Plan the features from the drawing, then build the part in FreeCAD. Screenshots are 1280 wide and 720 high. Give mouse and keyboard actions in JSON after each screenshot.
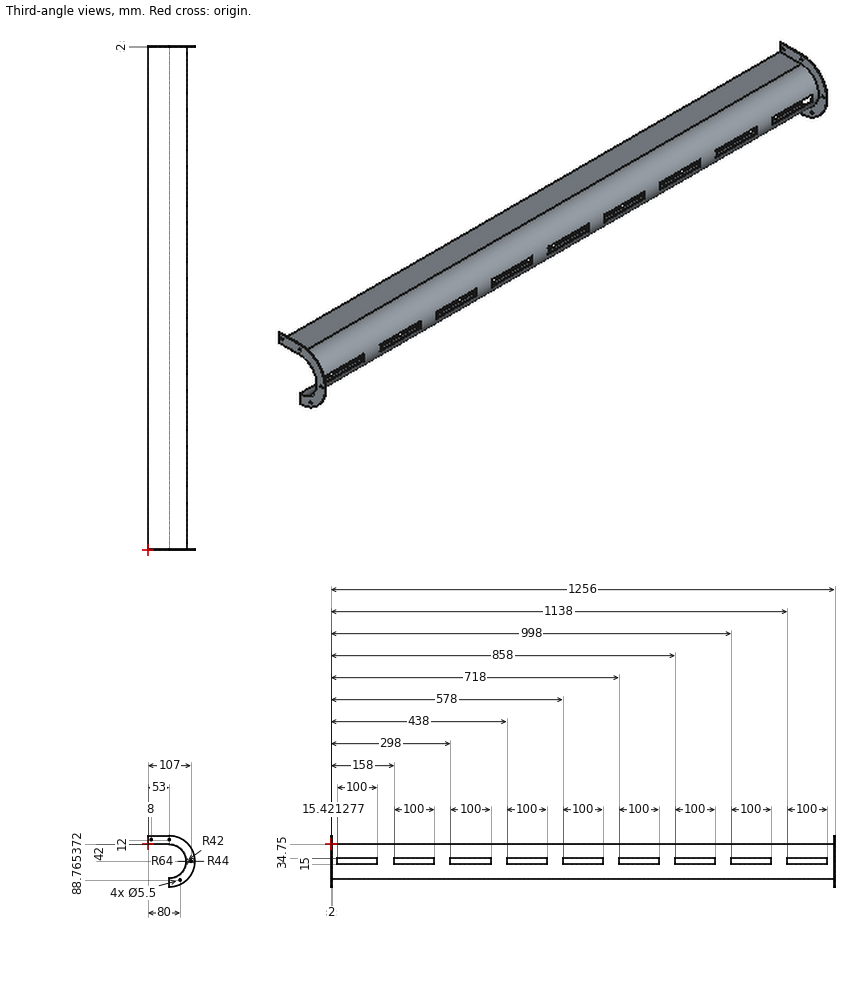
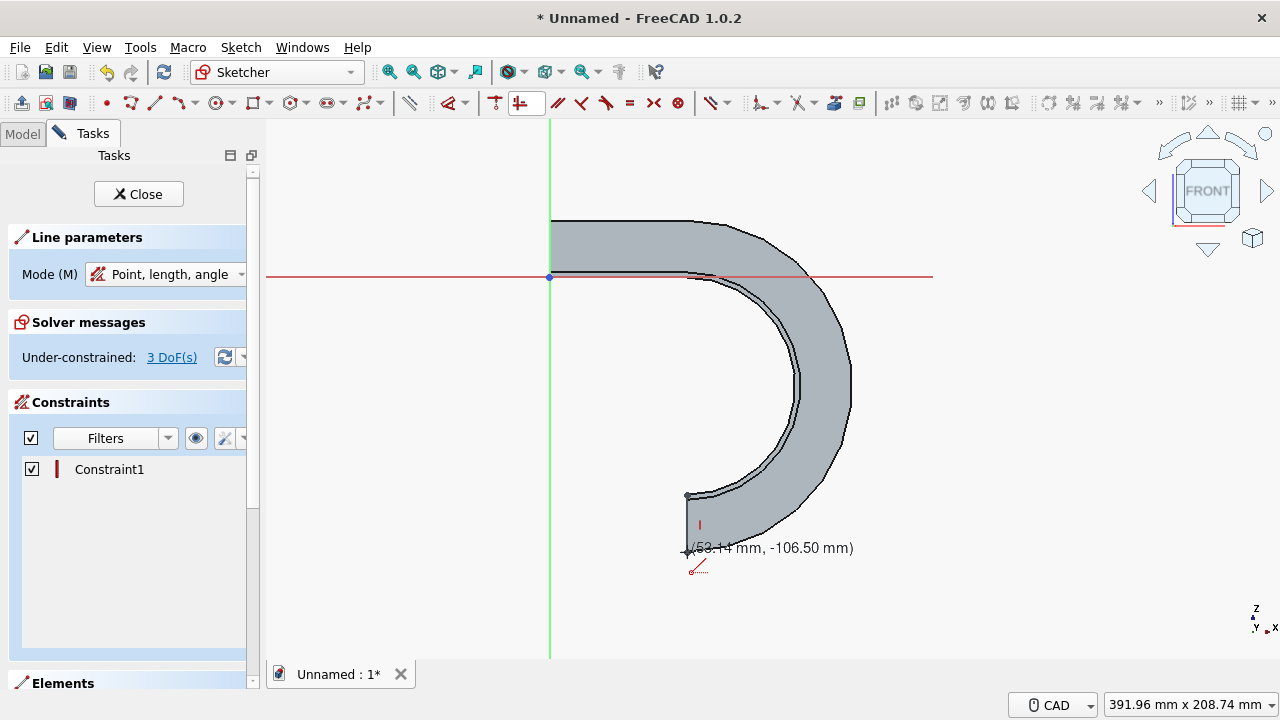
{"action": "left_click", "coordinate": [132, 104]}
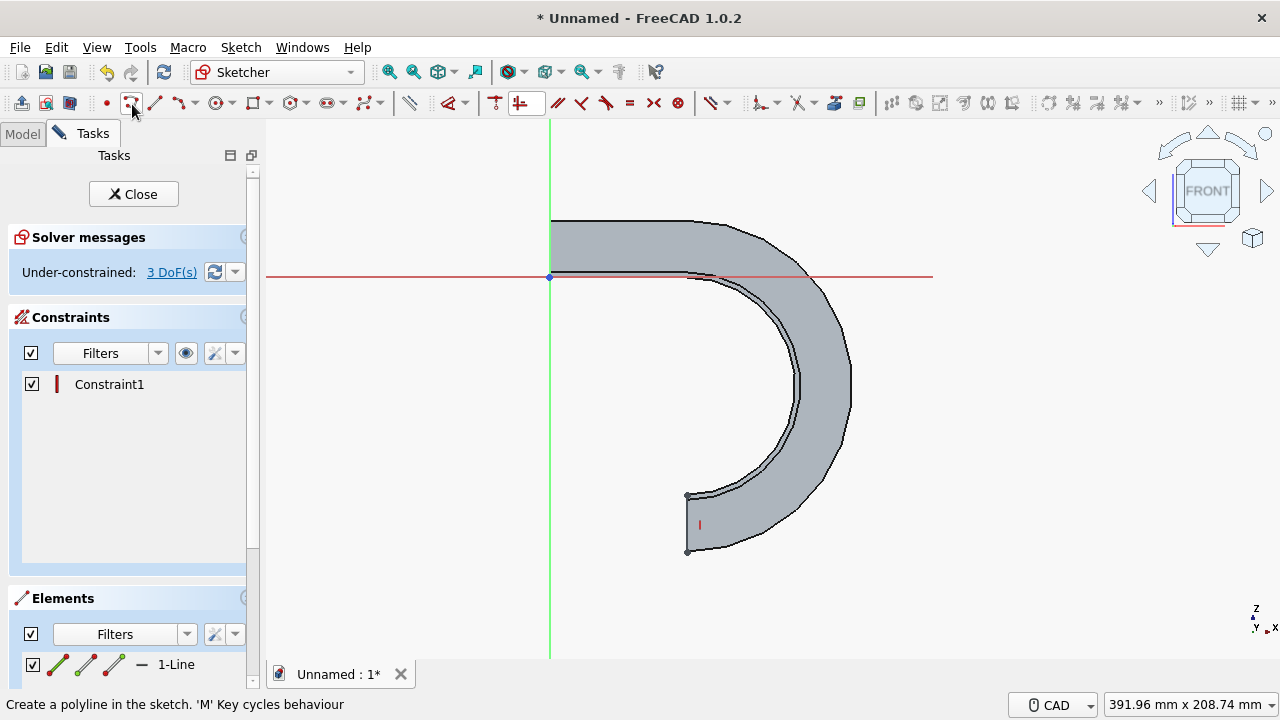
{"action": "left_click", "coordinate": [687, 221]}
{"action": "left_click", "coordinate": [550, 221]}
{"action": "left_click", "coordinate": [550, 277]}
{"action": "left_click", "coordinate": [687, 286]}
{"action": "right_click", "coordinate": [687, 286]}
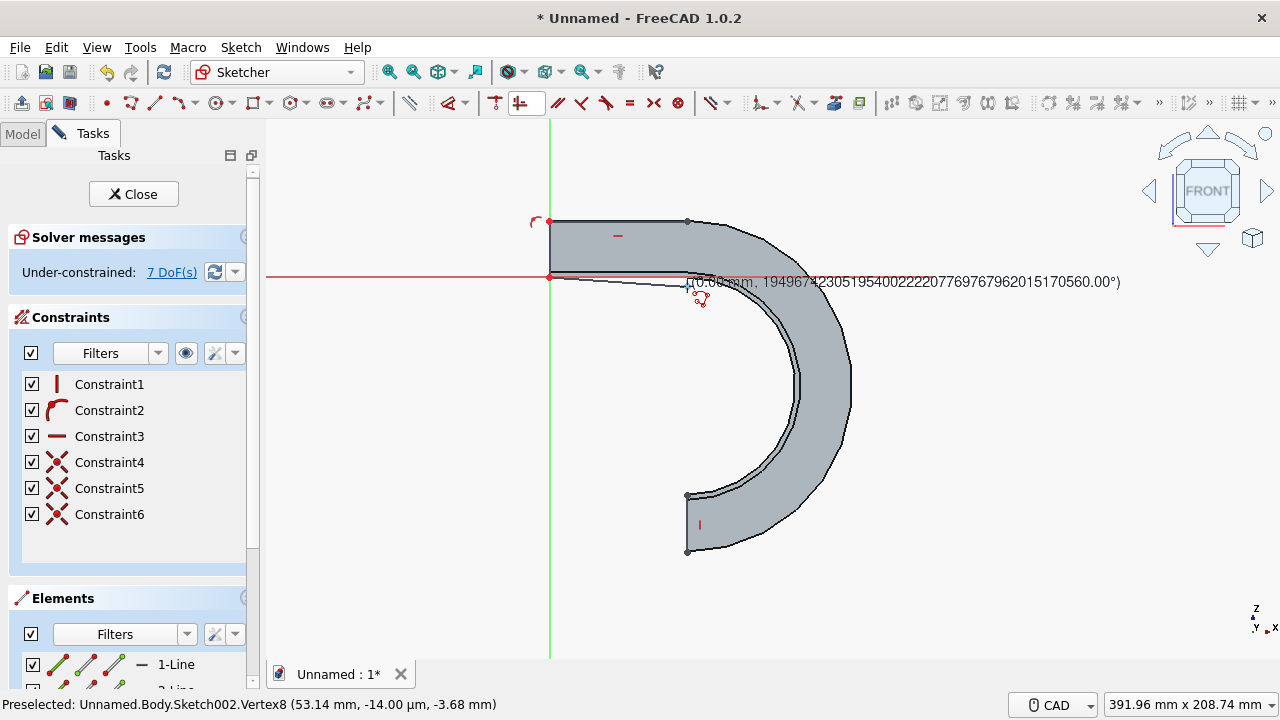
{"action": "left_click", "coordinate": [180, 104]}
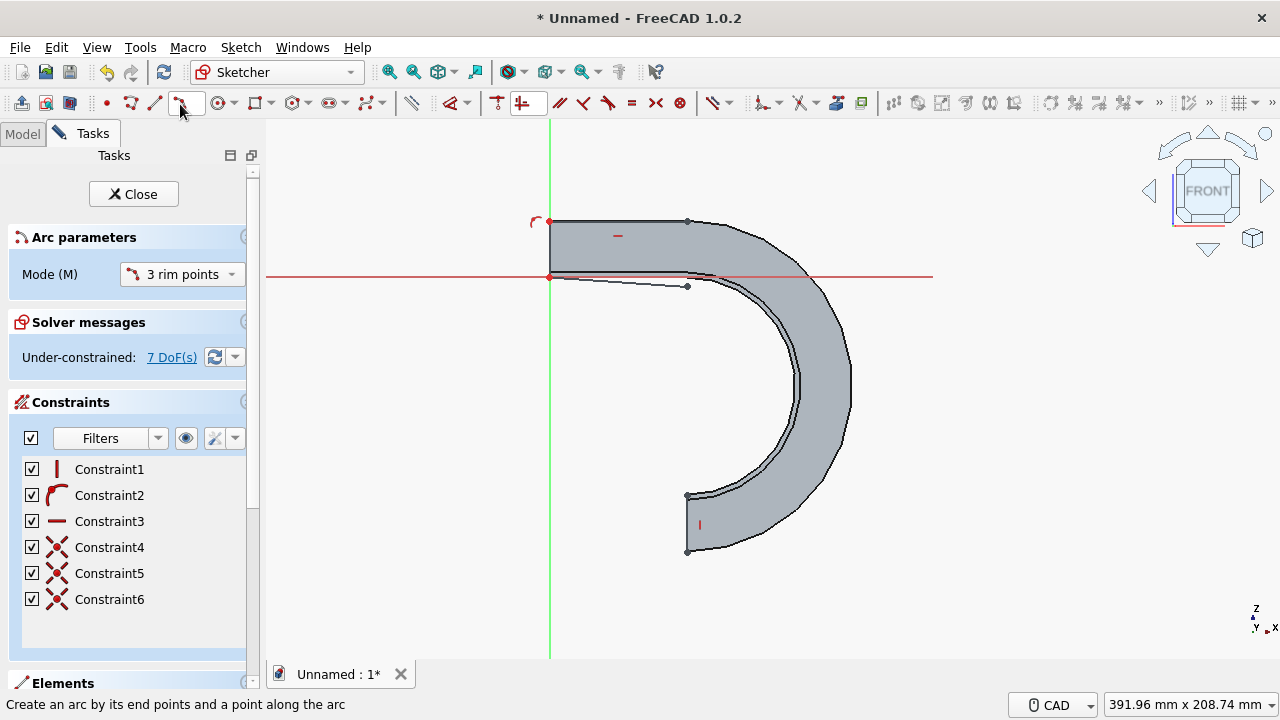
{"action": "left_click", "coordinate": [687, 553]}
{"action": "left_click", "coordinate": [687, 222]}
{"action": "left_click", "coordinate": [852, 386]}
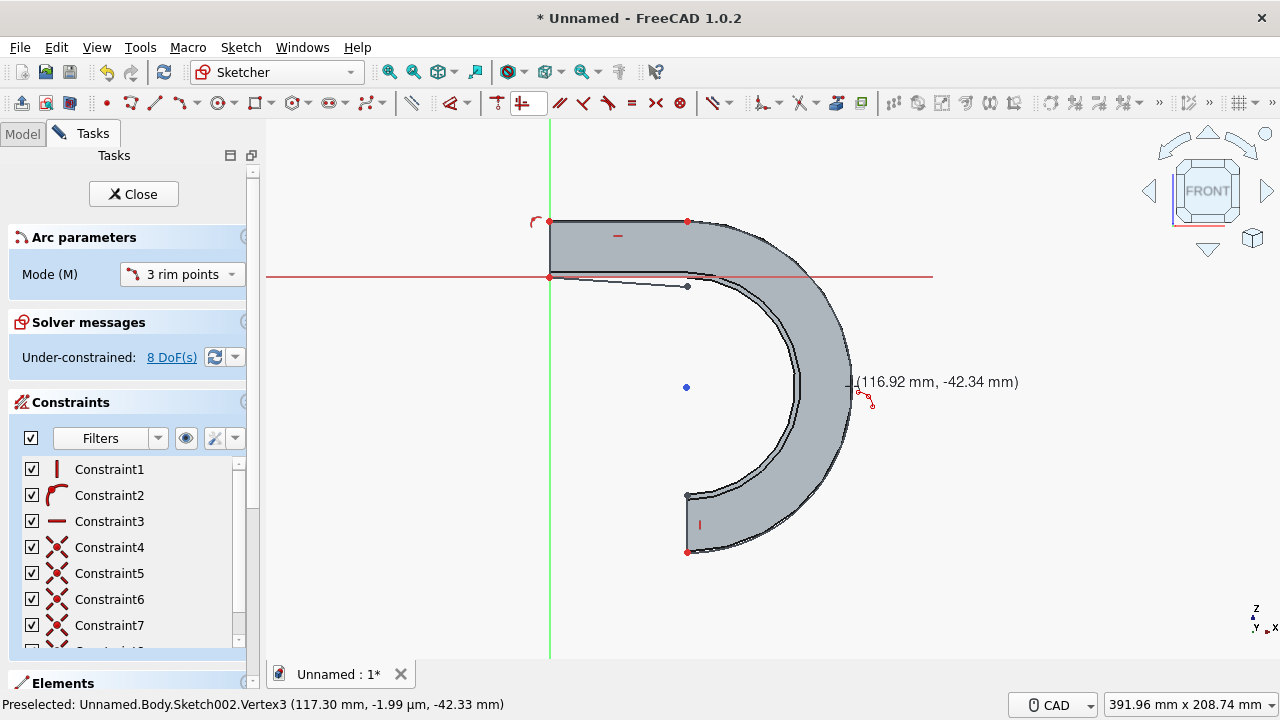
{"action": "left_click", "coordinate": [687, 287]}
{"action": "left_click", "coordinate": [687, 496]}
{"action": "left_click", "coordinate": [795, 386]}
{"action": "key", "text": "Escape"}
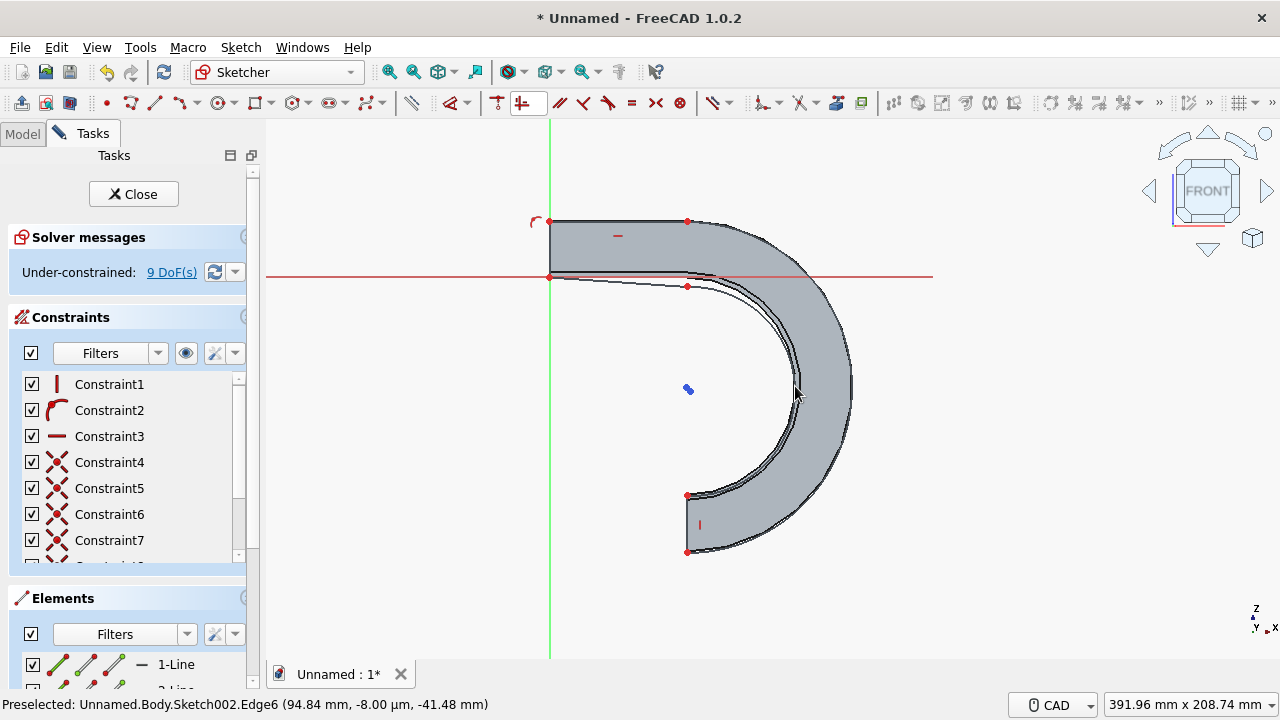
{"action": "left_click", "coordinate": [591, 280]}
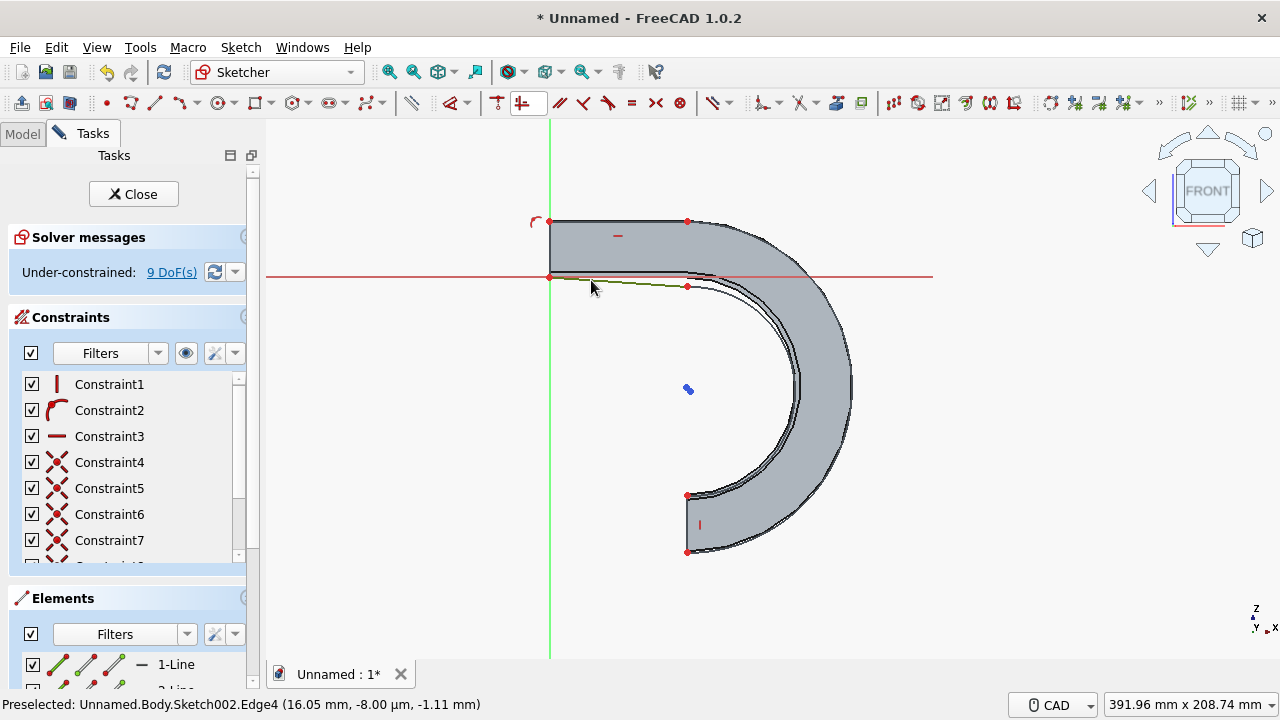
{"action": "left_click", "coordinate": [774, 454]}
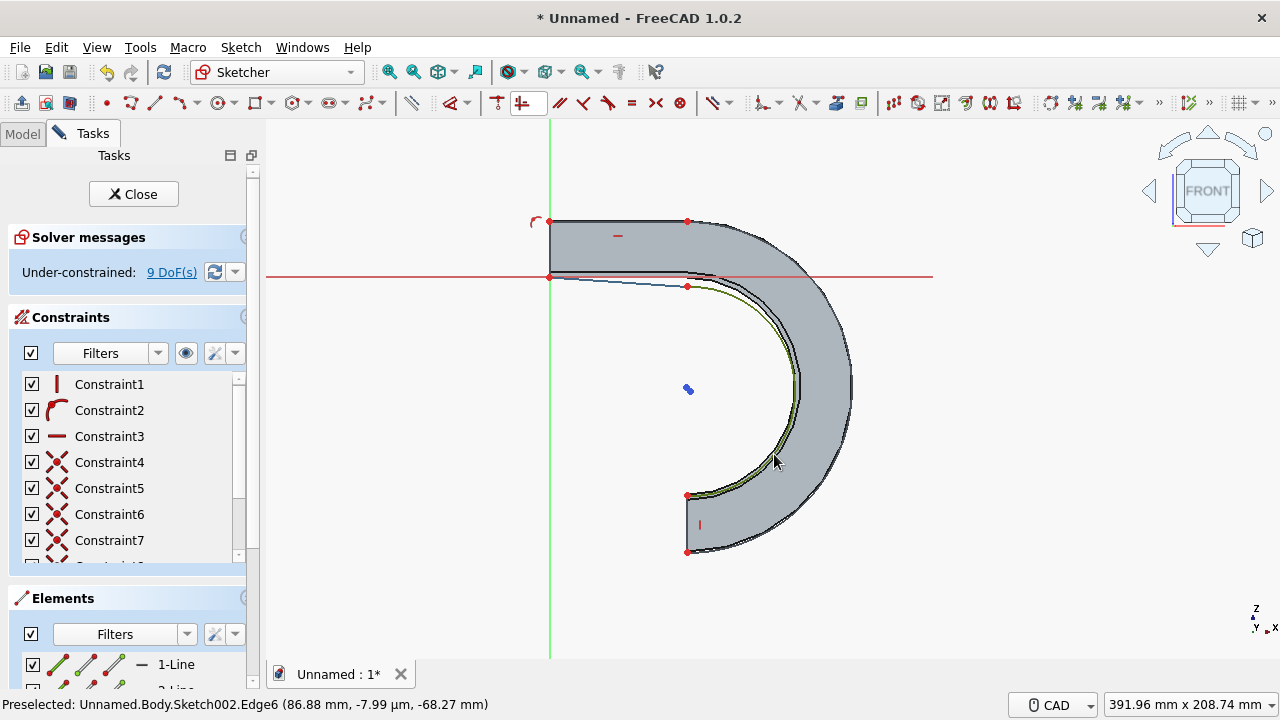
{"action": "key", "text": "t"}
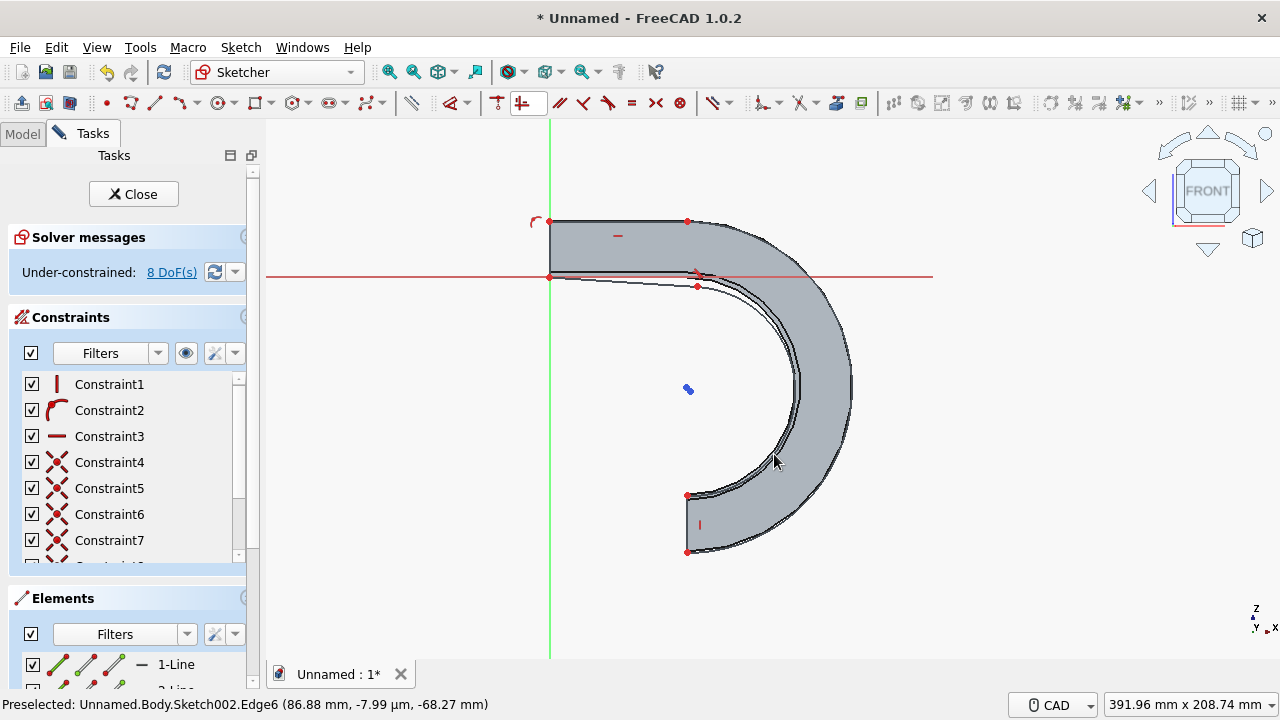
{"action": "left_click", "coordinate": [594, 280]}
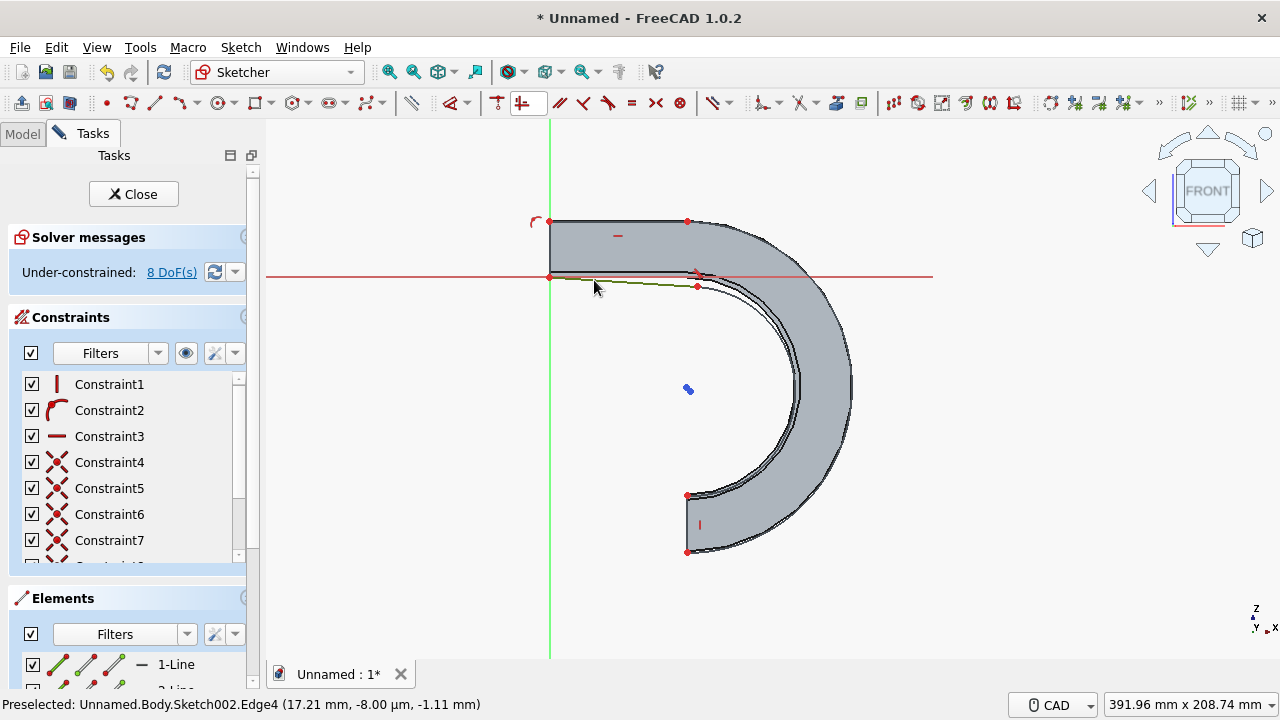
{"action": "left_click", "coordinate": [542, 104]}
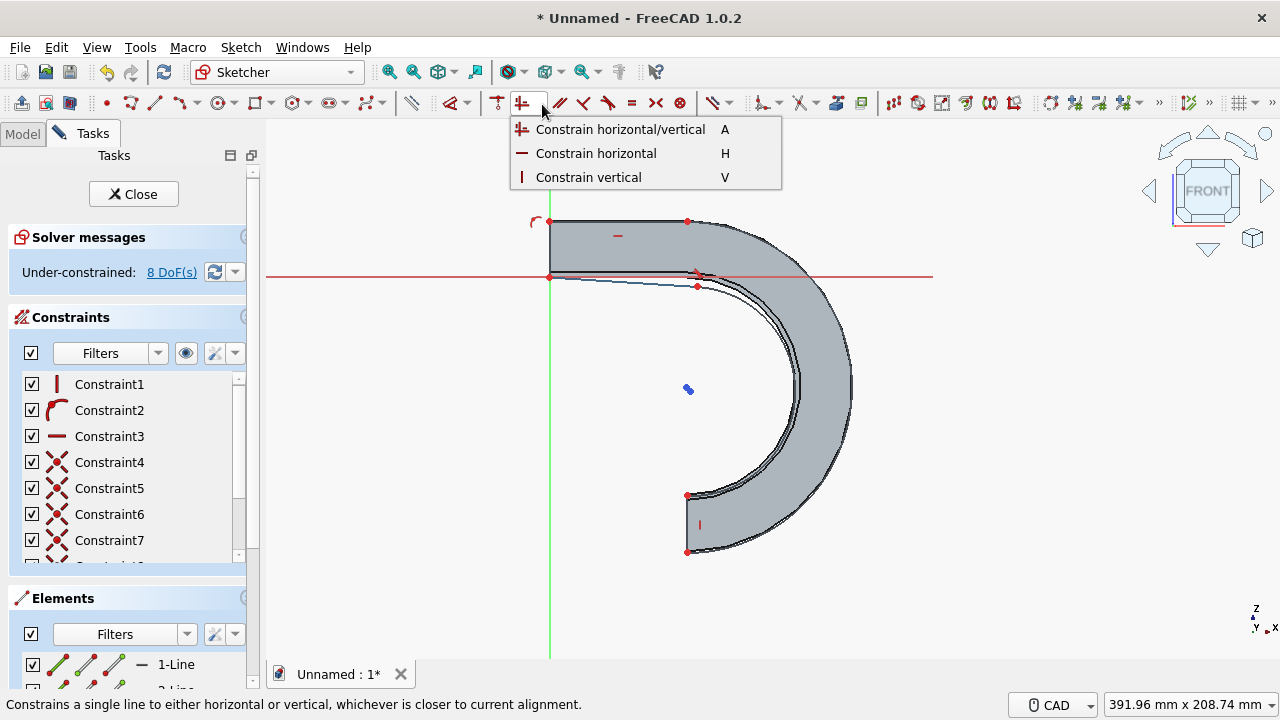
{"action": "left_click", "coordinate": [646, 153]}